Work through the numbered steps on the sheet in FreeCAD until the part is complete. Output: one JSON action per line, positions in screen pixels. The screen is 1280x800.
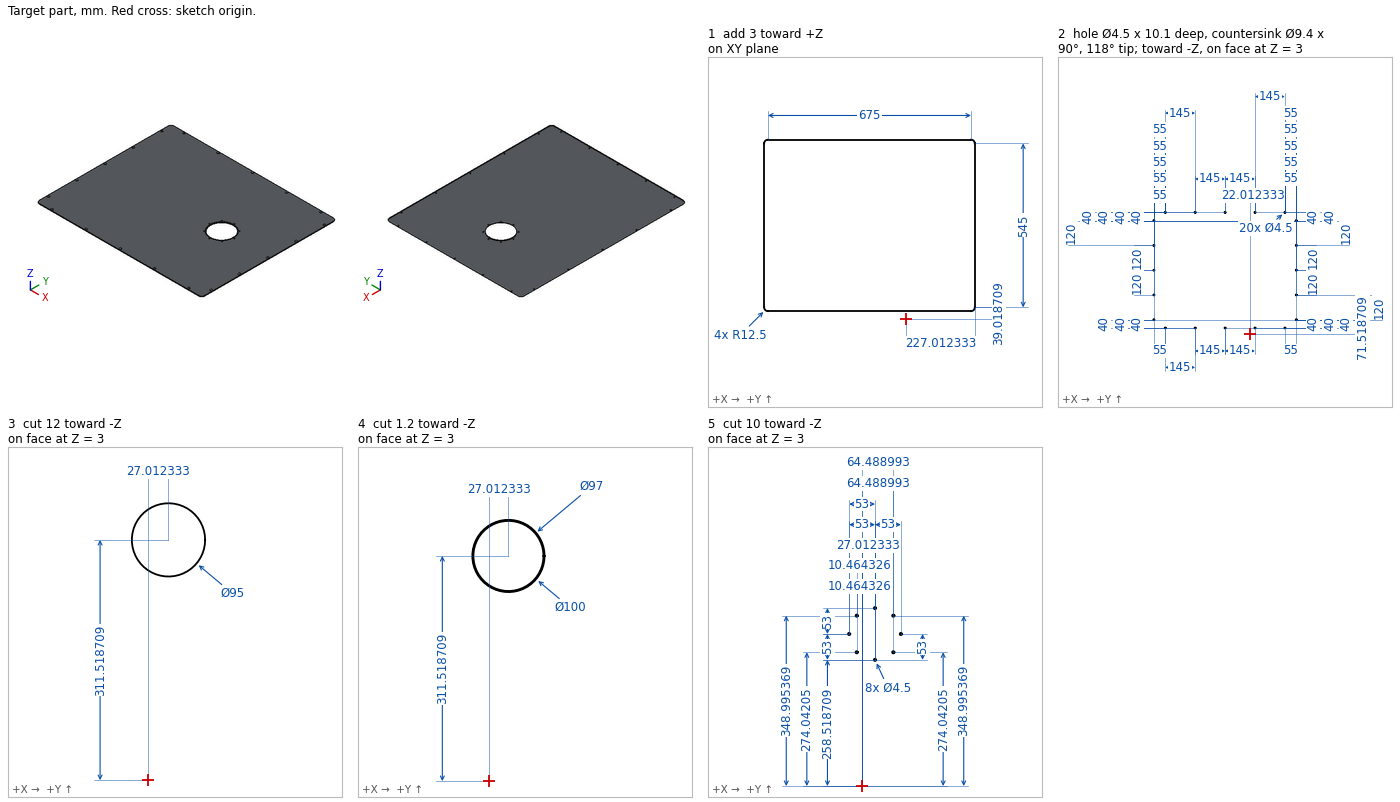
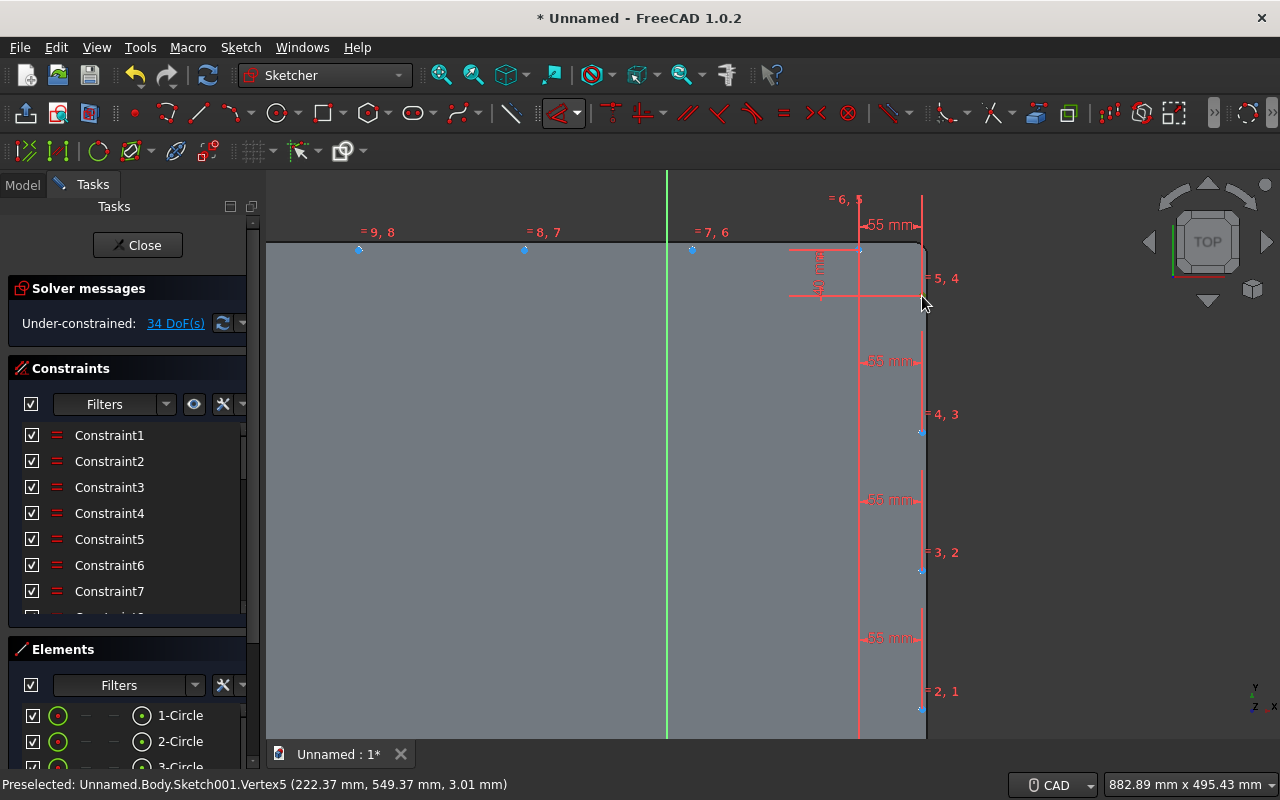
{"action": "left_click", "coordinate": [693, 250]}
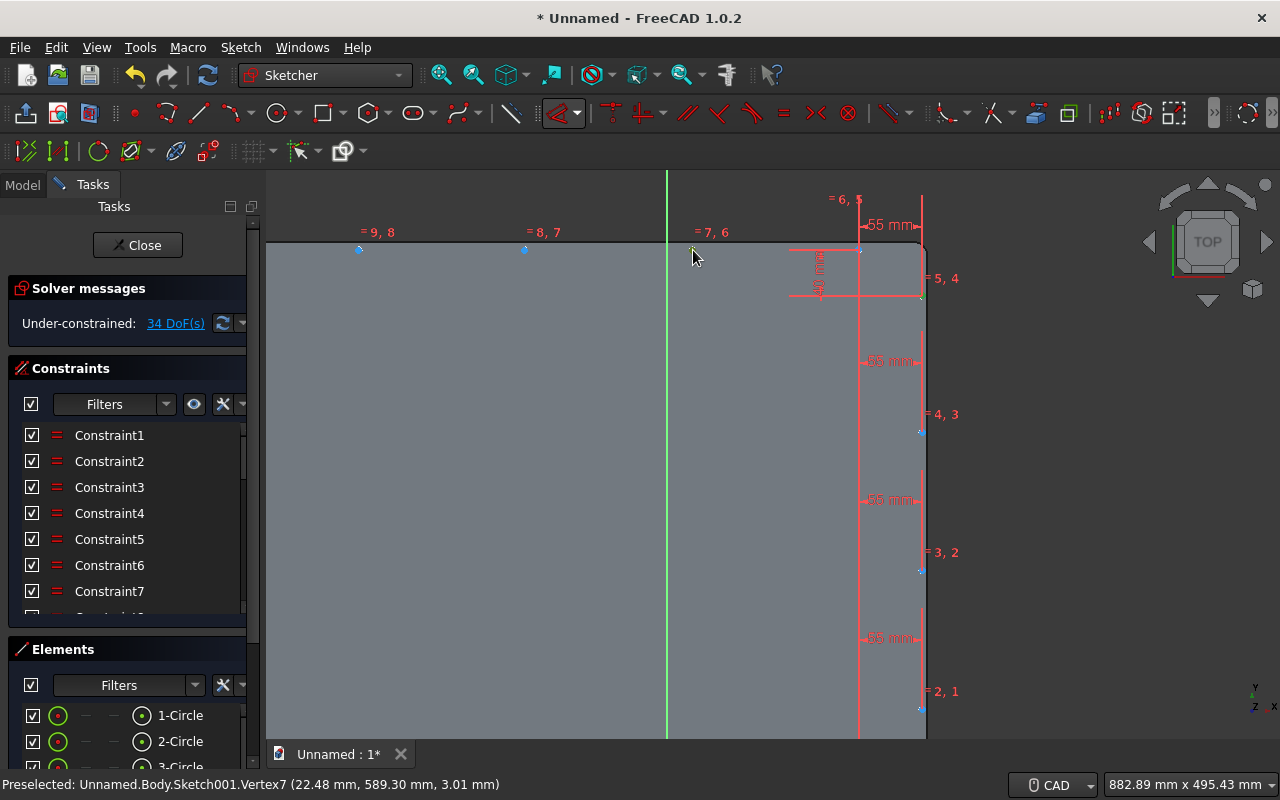
{"action": "key", "text": "i"}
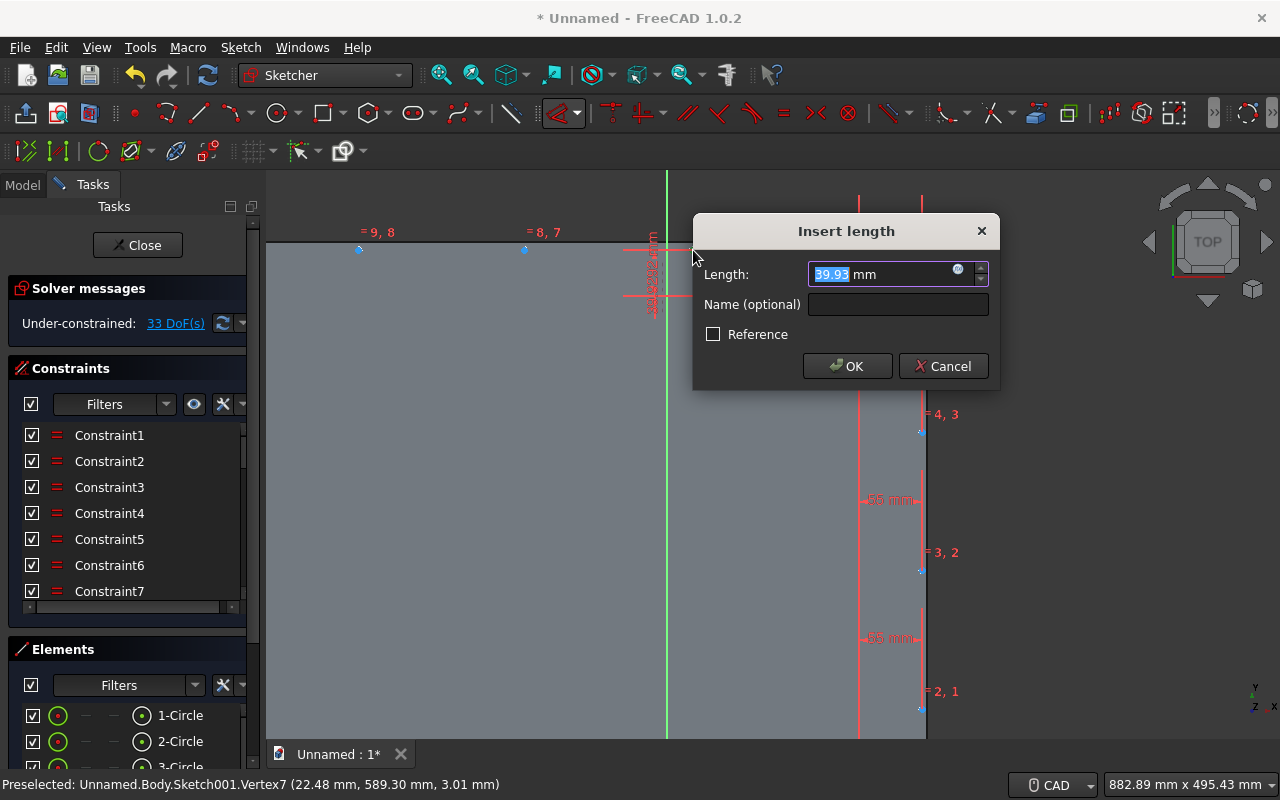
{"action": "type", "text": "40"}
{"action": "key", "text": "Return"}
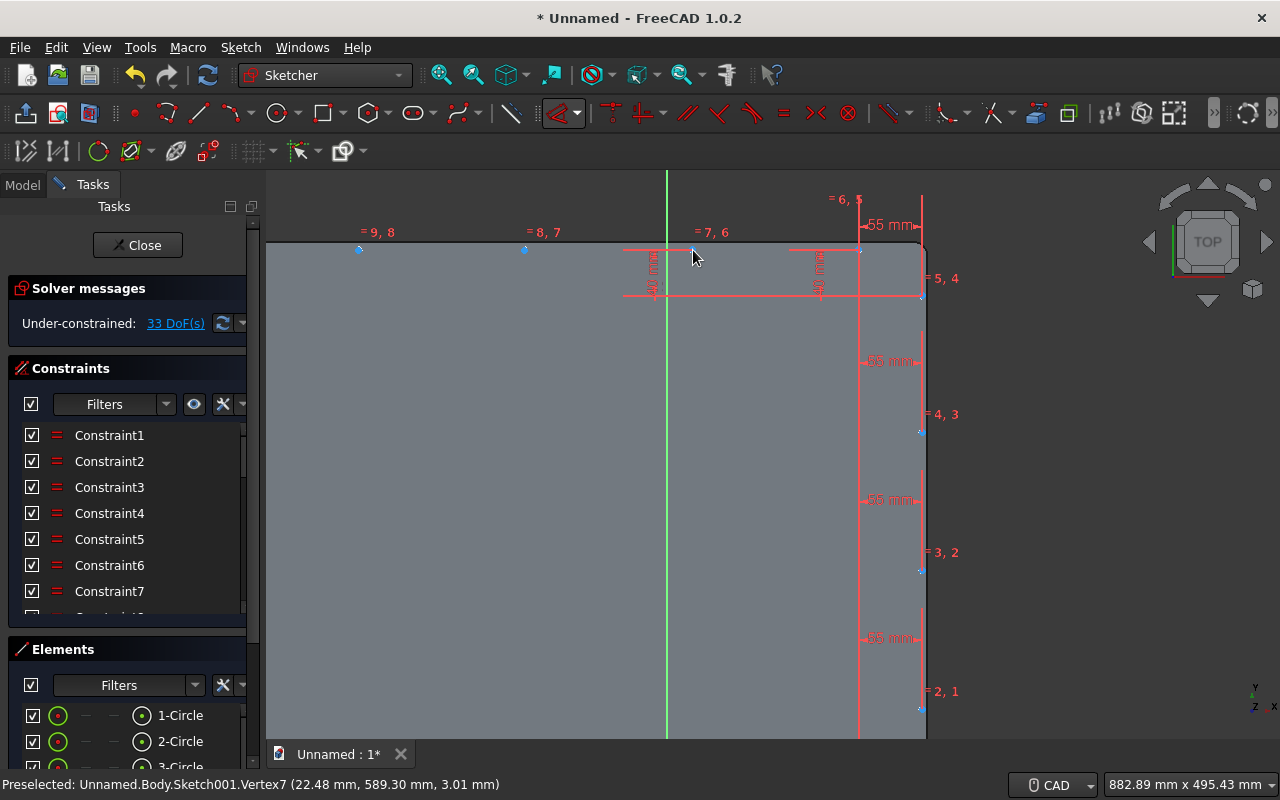
{"action": "left_click", "coordinate": [922, 296]}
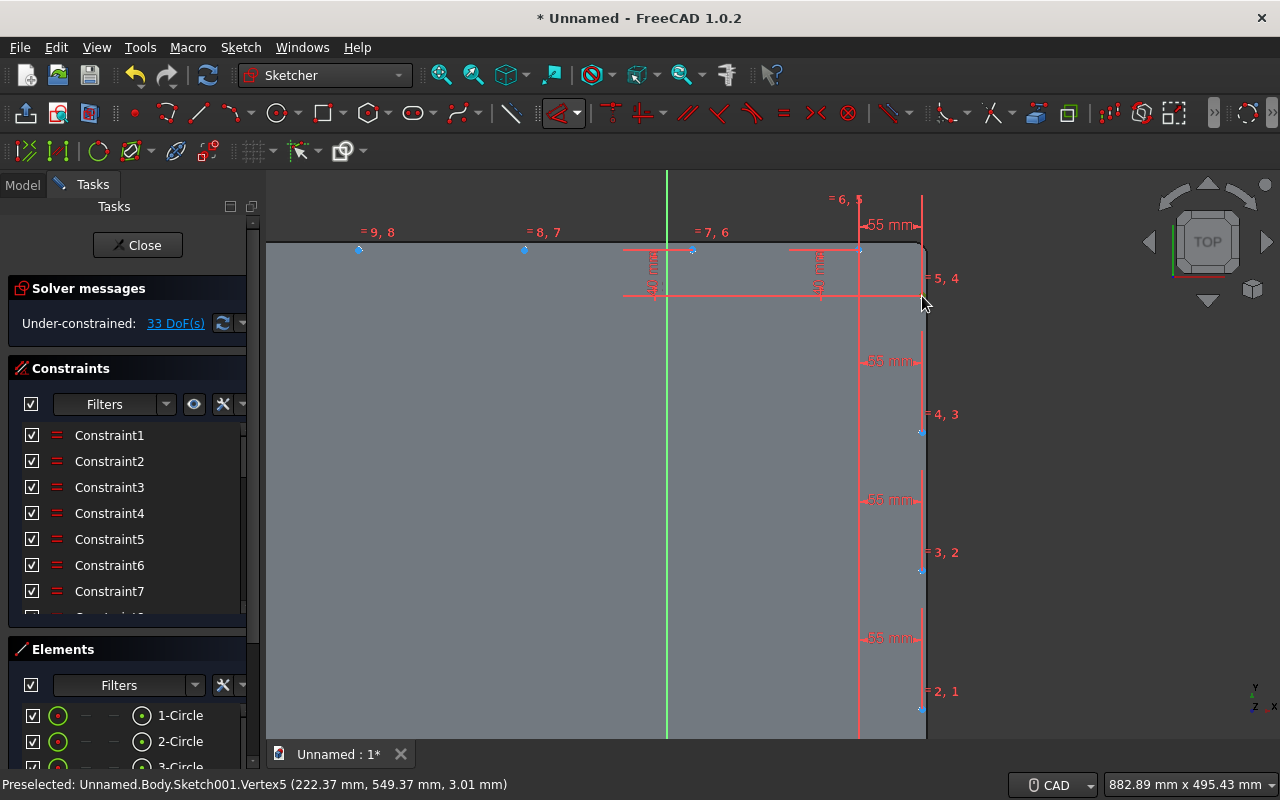
{"action": "left_click", "coordinate": [525, 250]}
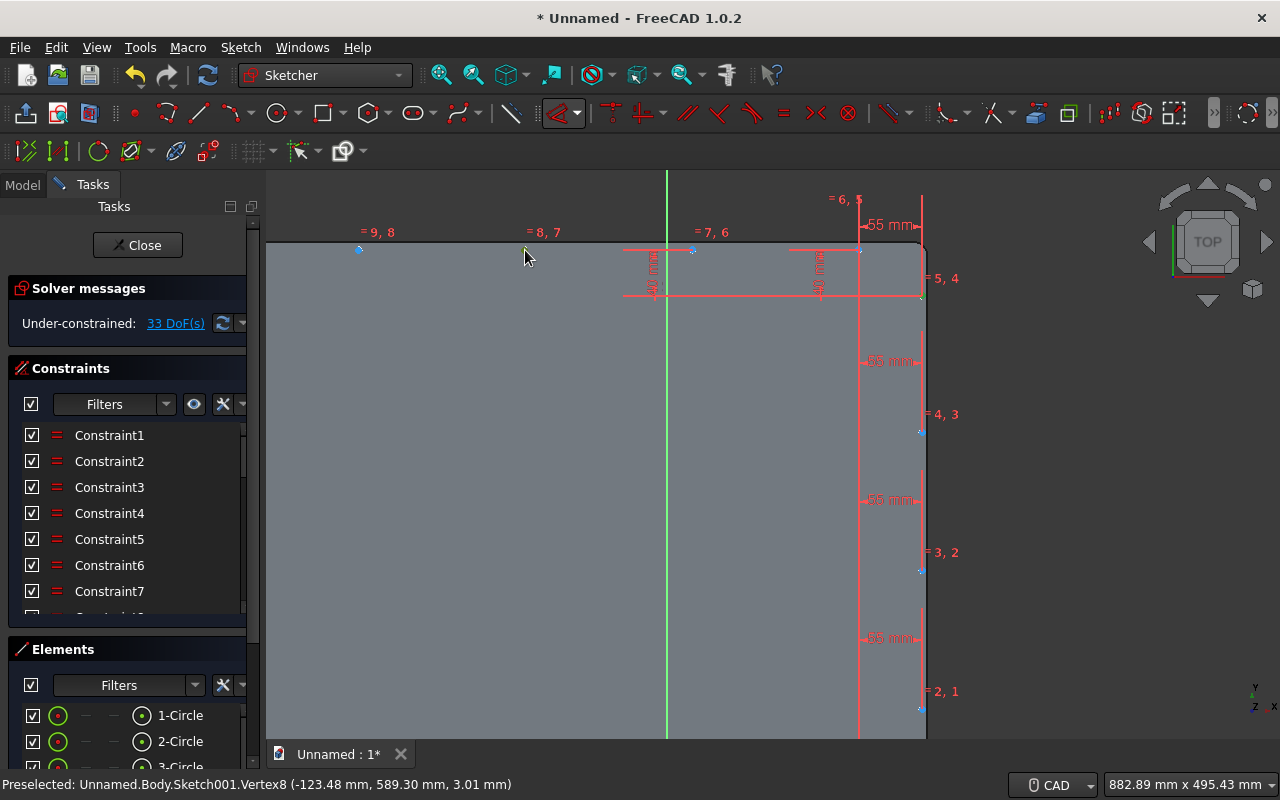
{"action": "key", "text": "i"}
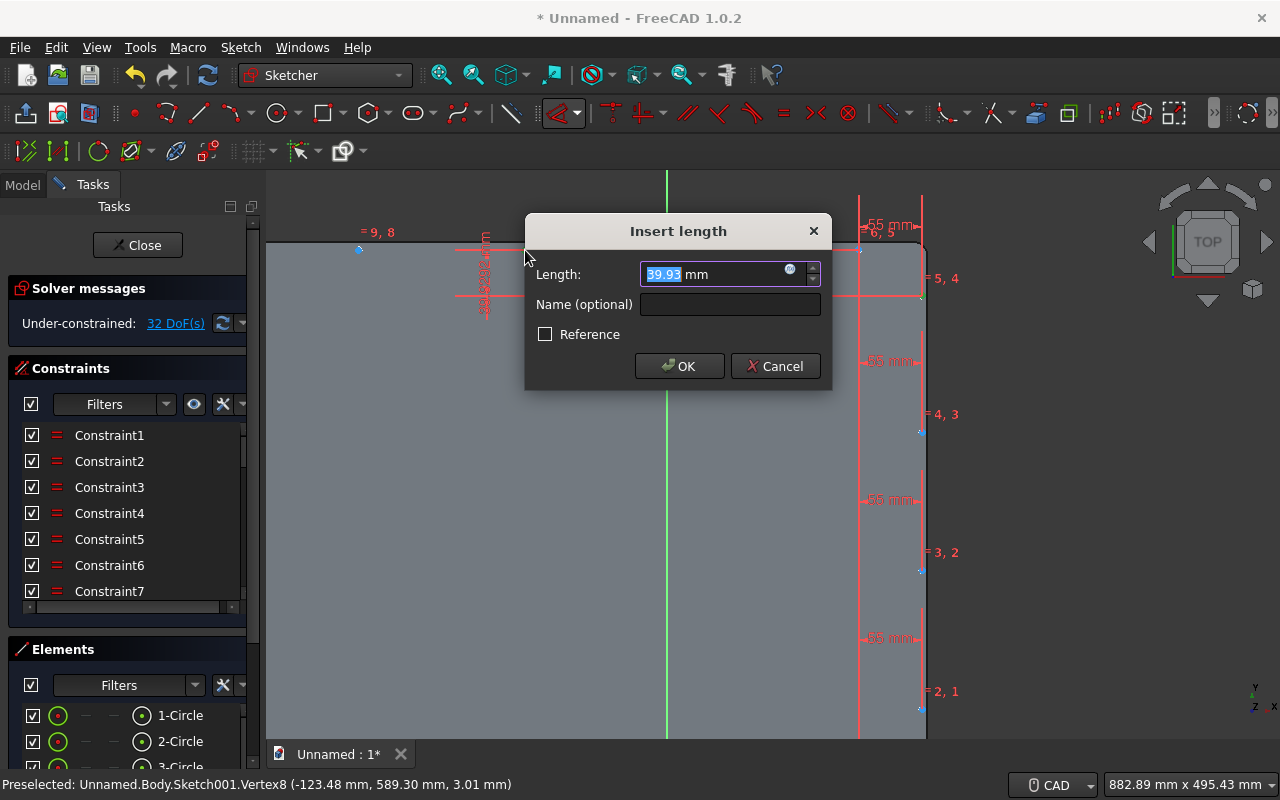
{"action": "type", "text": "40"}
{"action": "key", "text": "Return"}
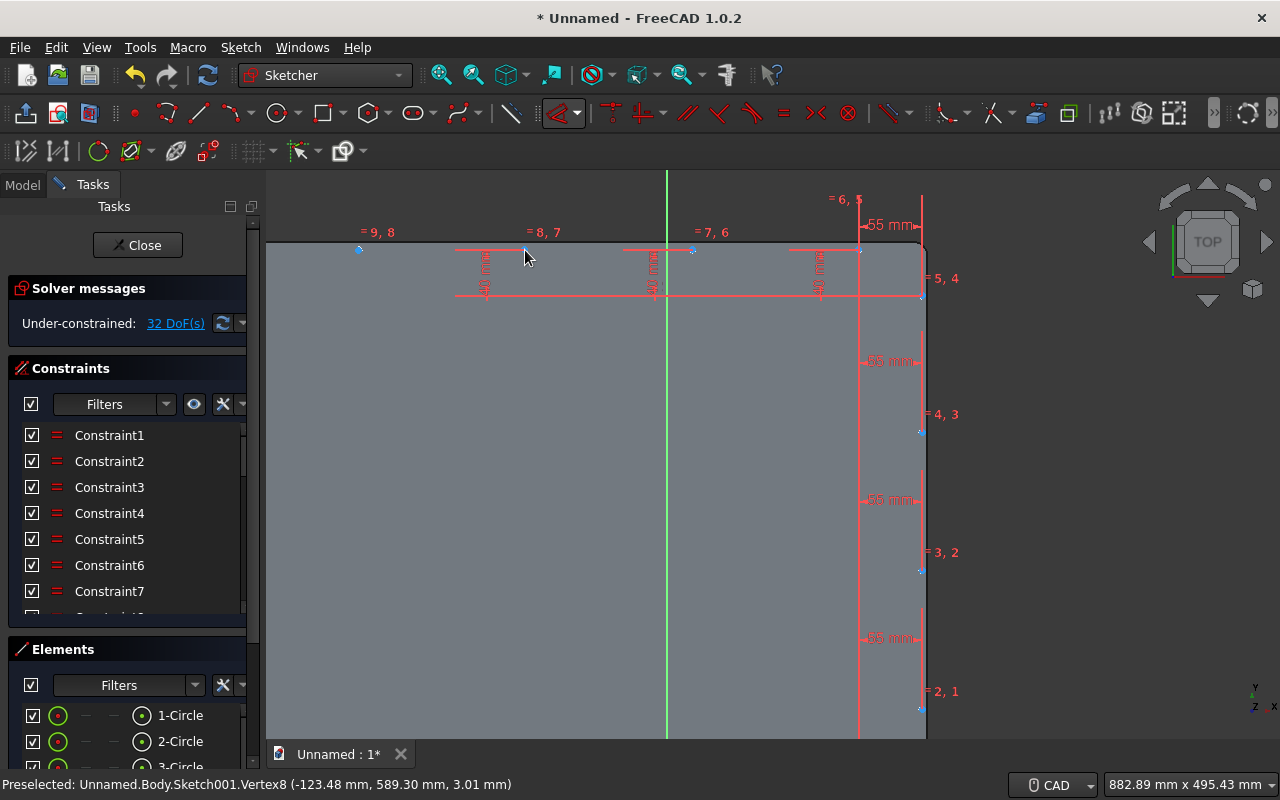
{"action": "left_click", "coordinate": [922, 296]}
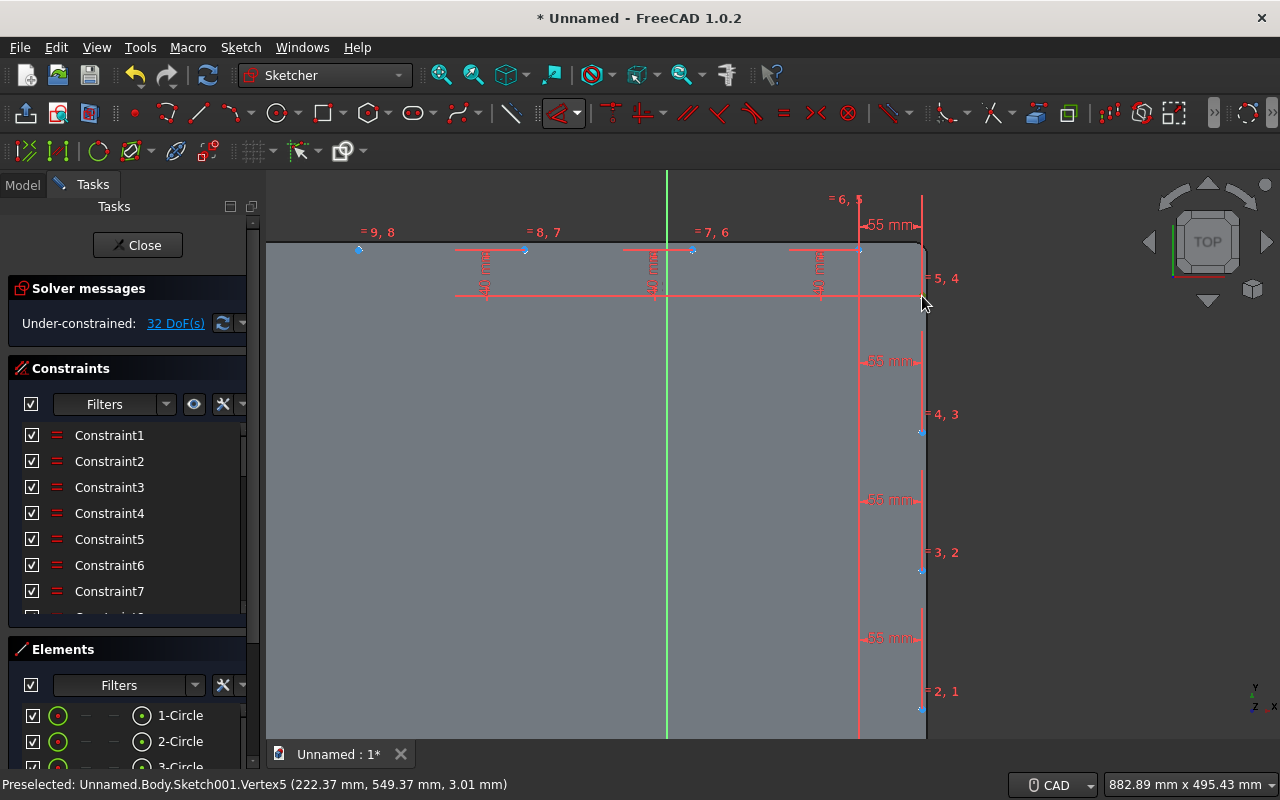
{"action": "left_click", "coordinate": [359, 250]}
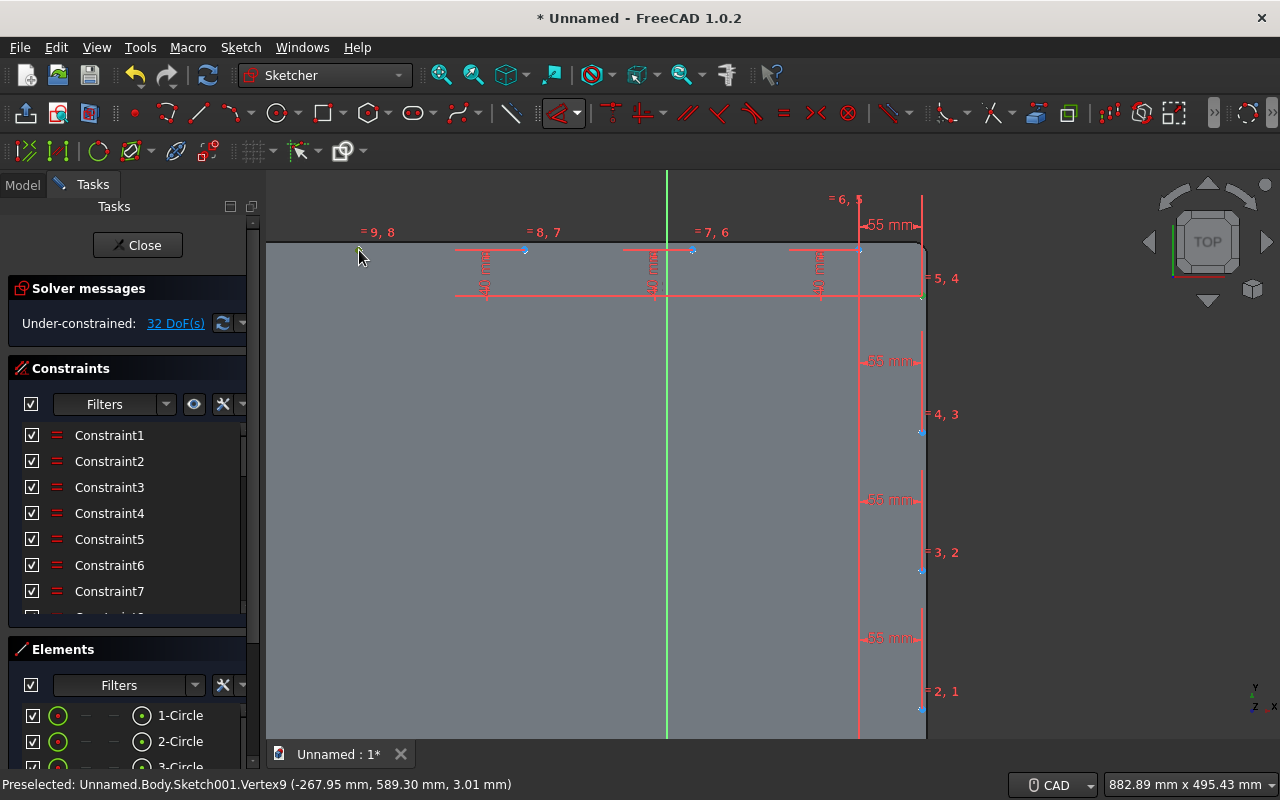
{"action": "key", "text": "i"}